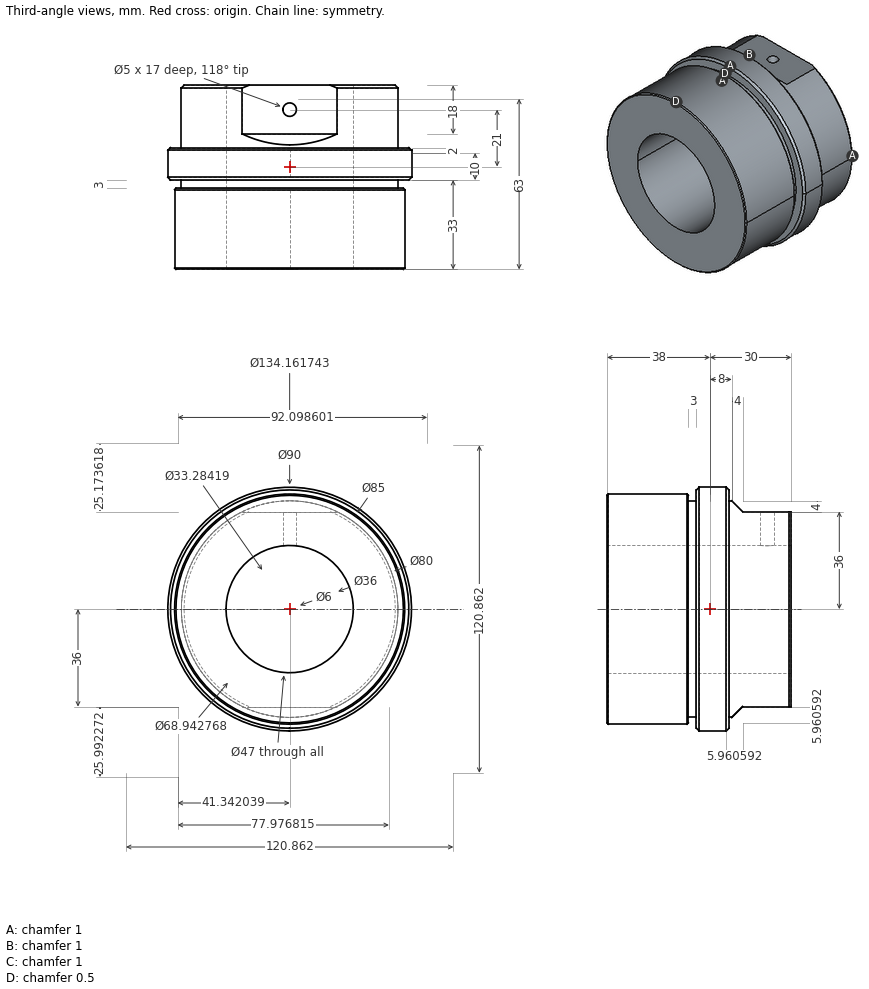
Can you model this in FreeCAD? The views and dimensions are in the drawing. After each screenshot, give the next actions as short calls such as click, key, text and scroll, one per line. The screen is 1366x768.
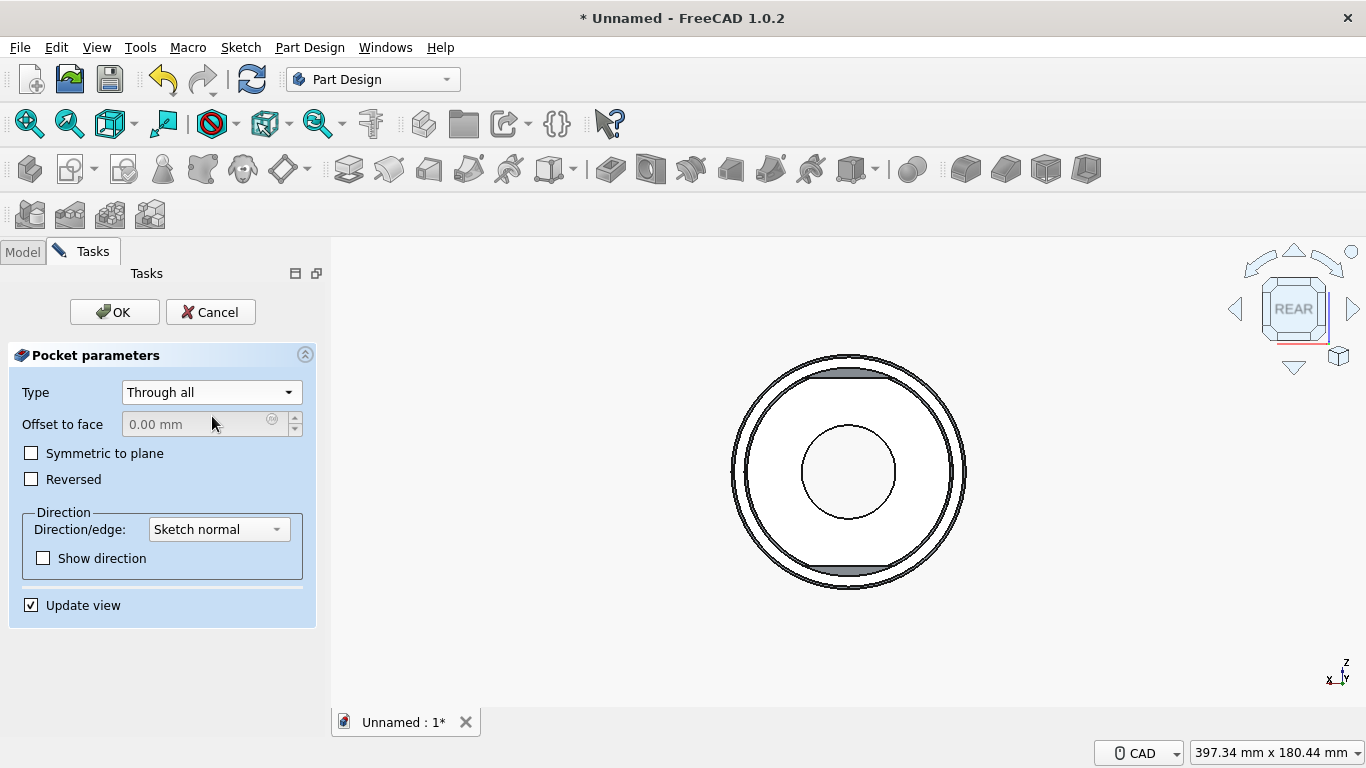
click(30, 479)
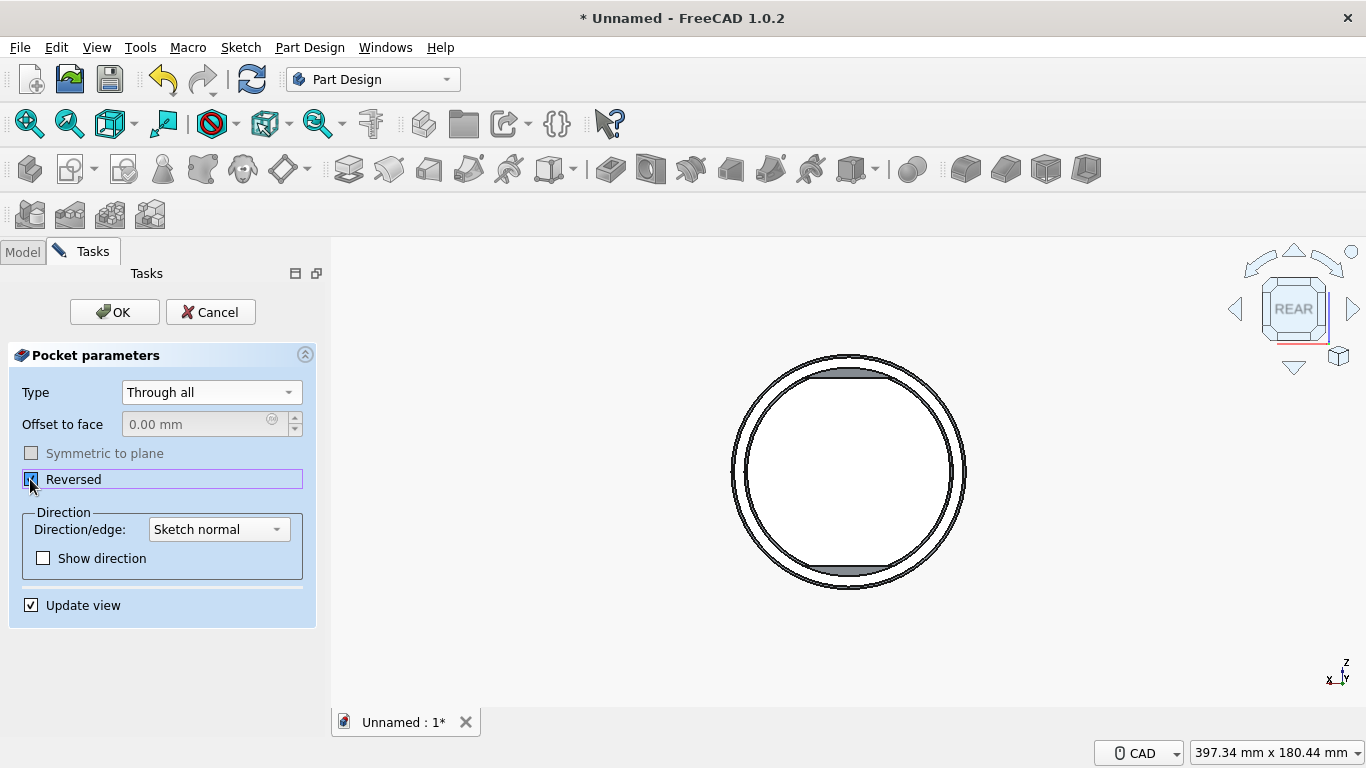
click(115, 312)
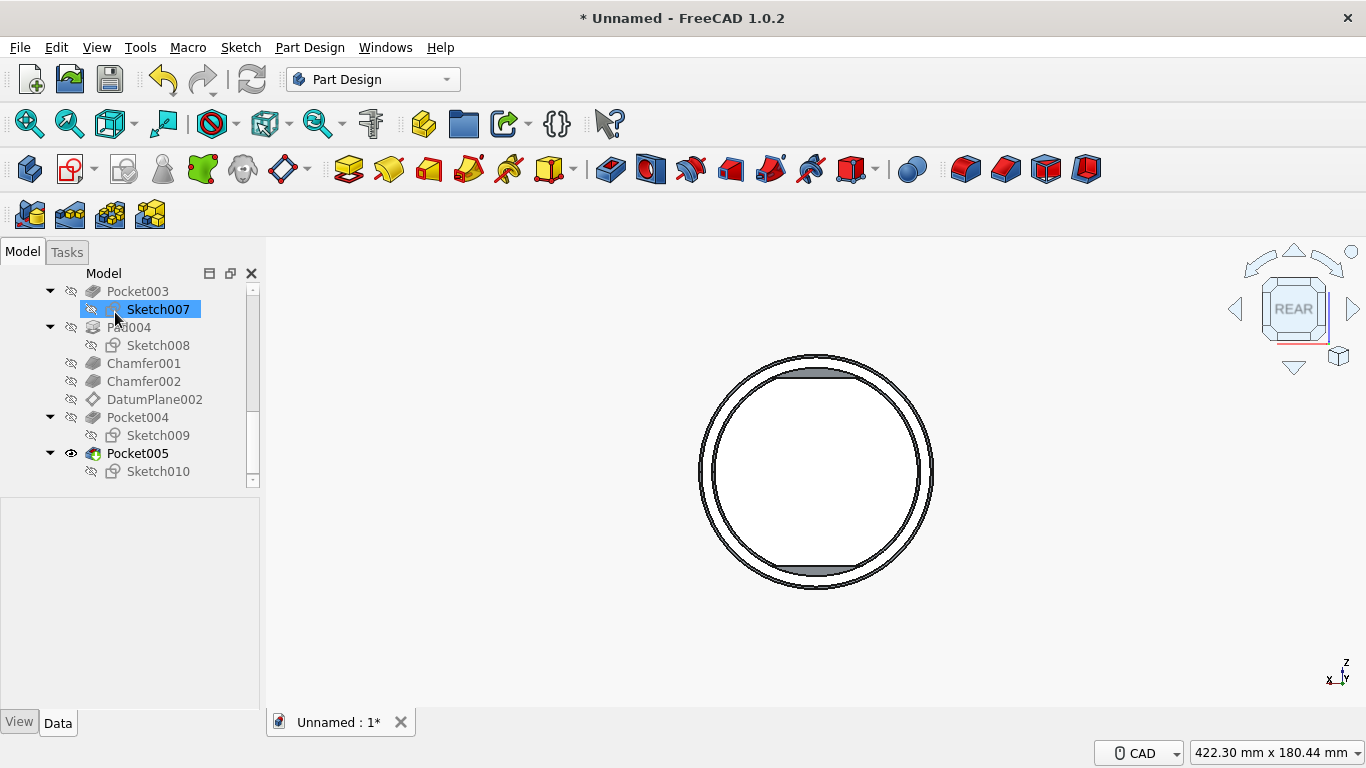
click(816, 471)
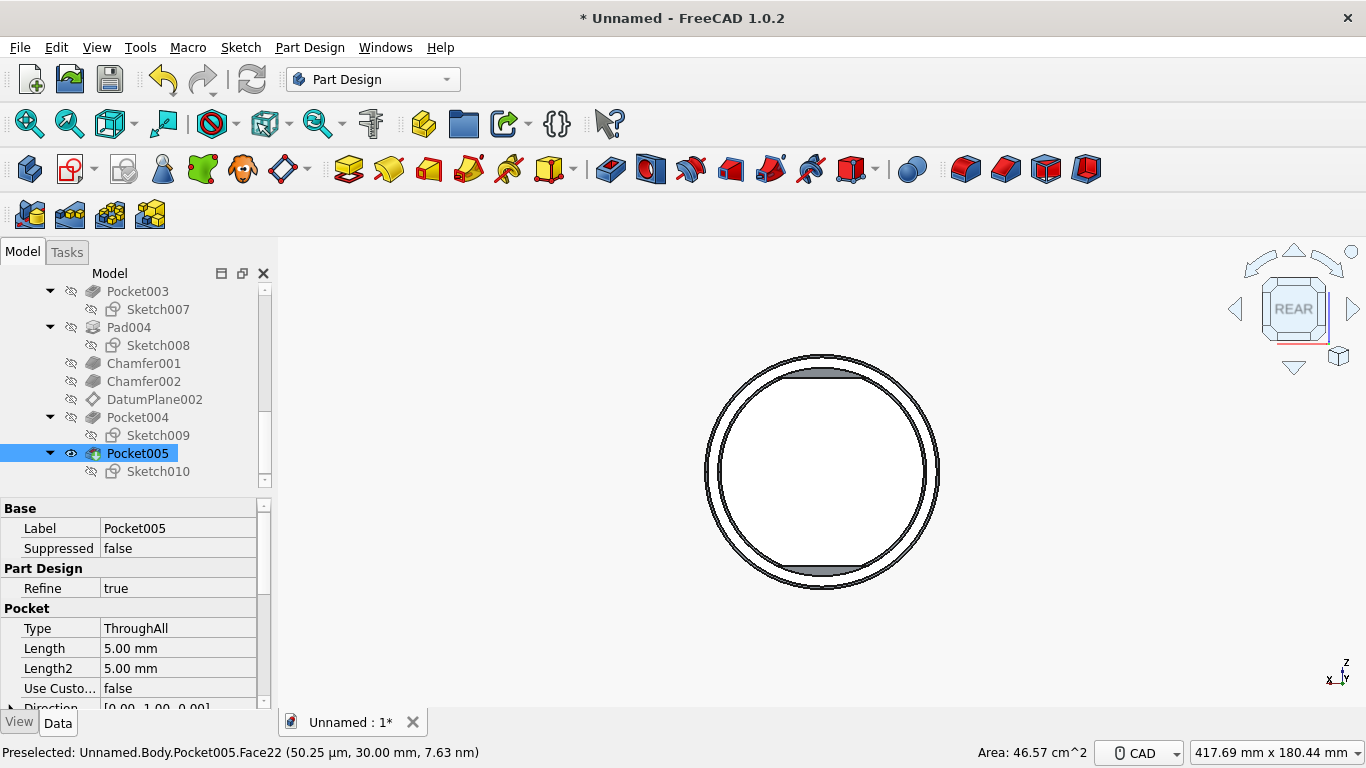
click(70, 170)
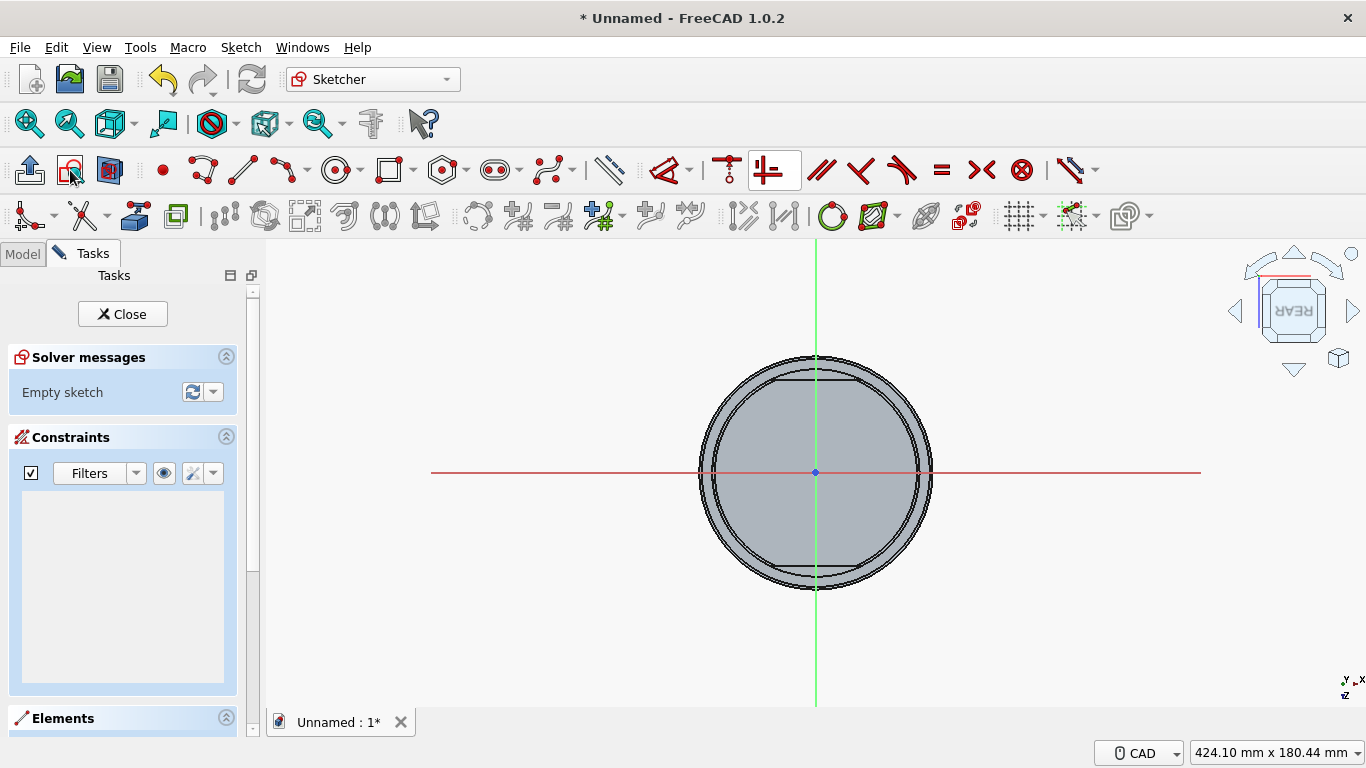
scroll(872, 473, up, 4)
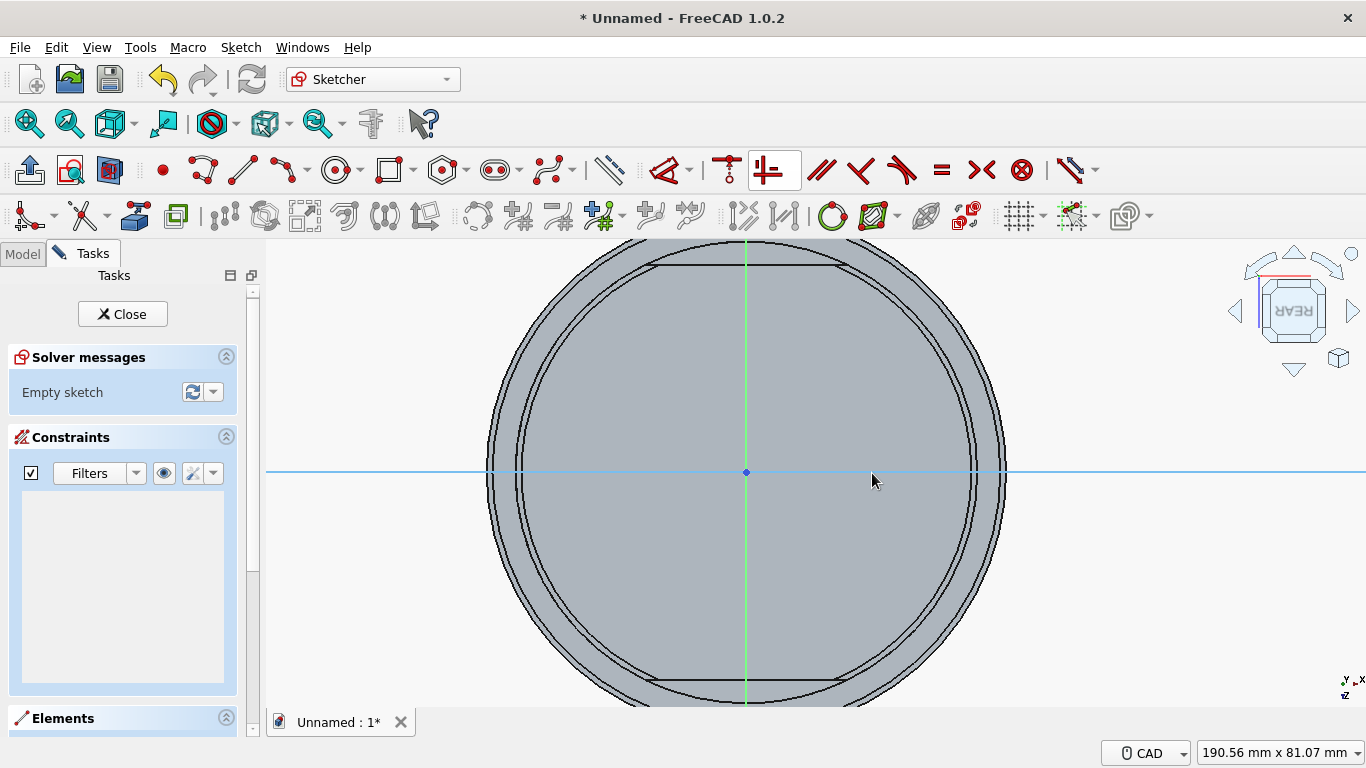
click(336, 170)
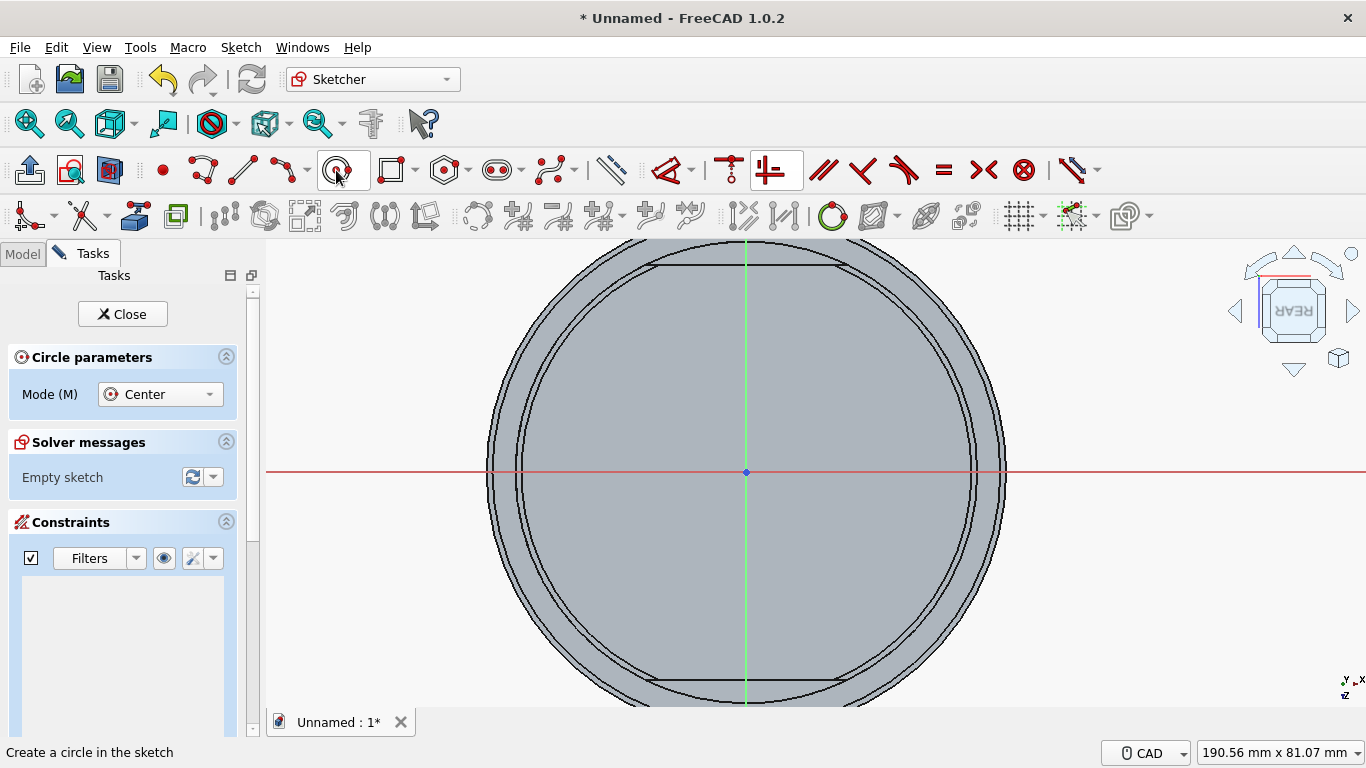
click(746, 472)
click(842, 376)
key(Escape)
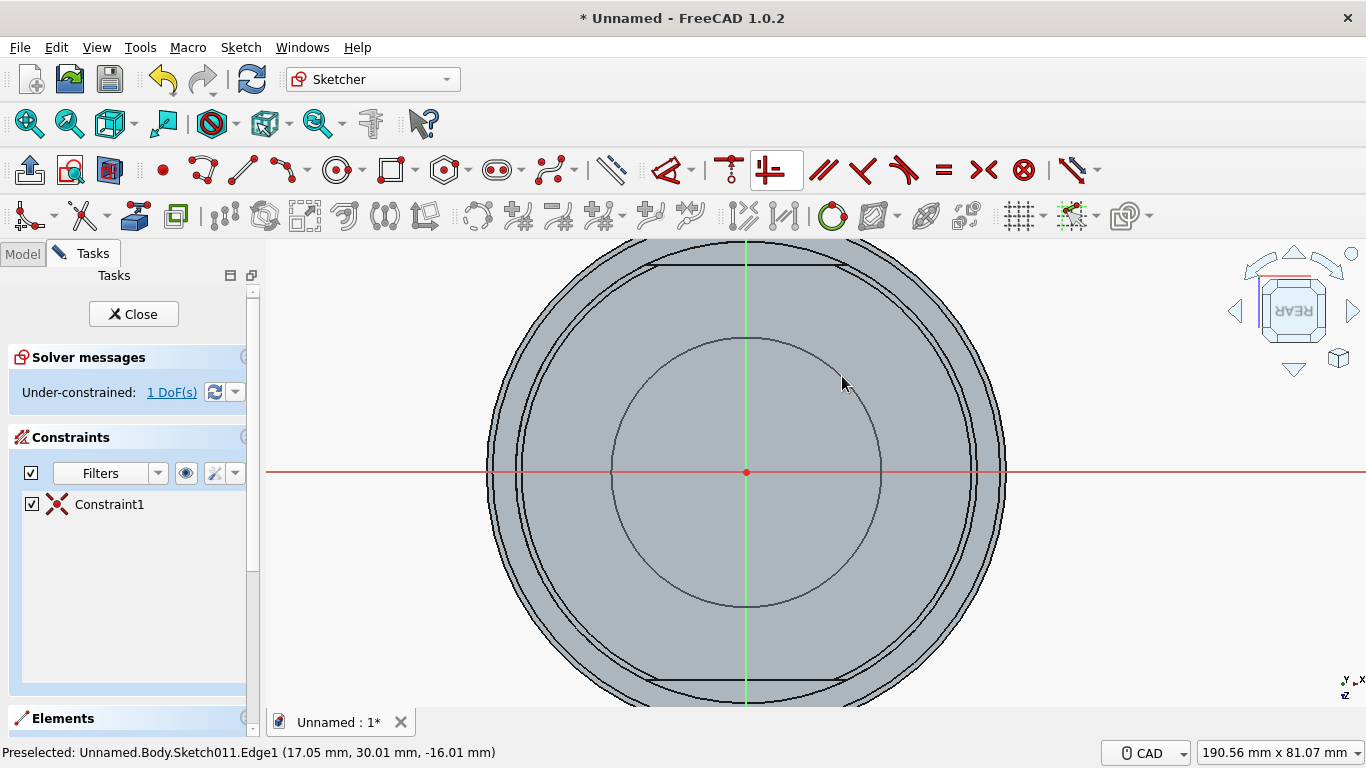
click(666, 170)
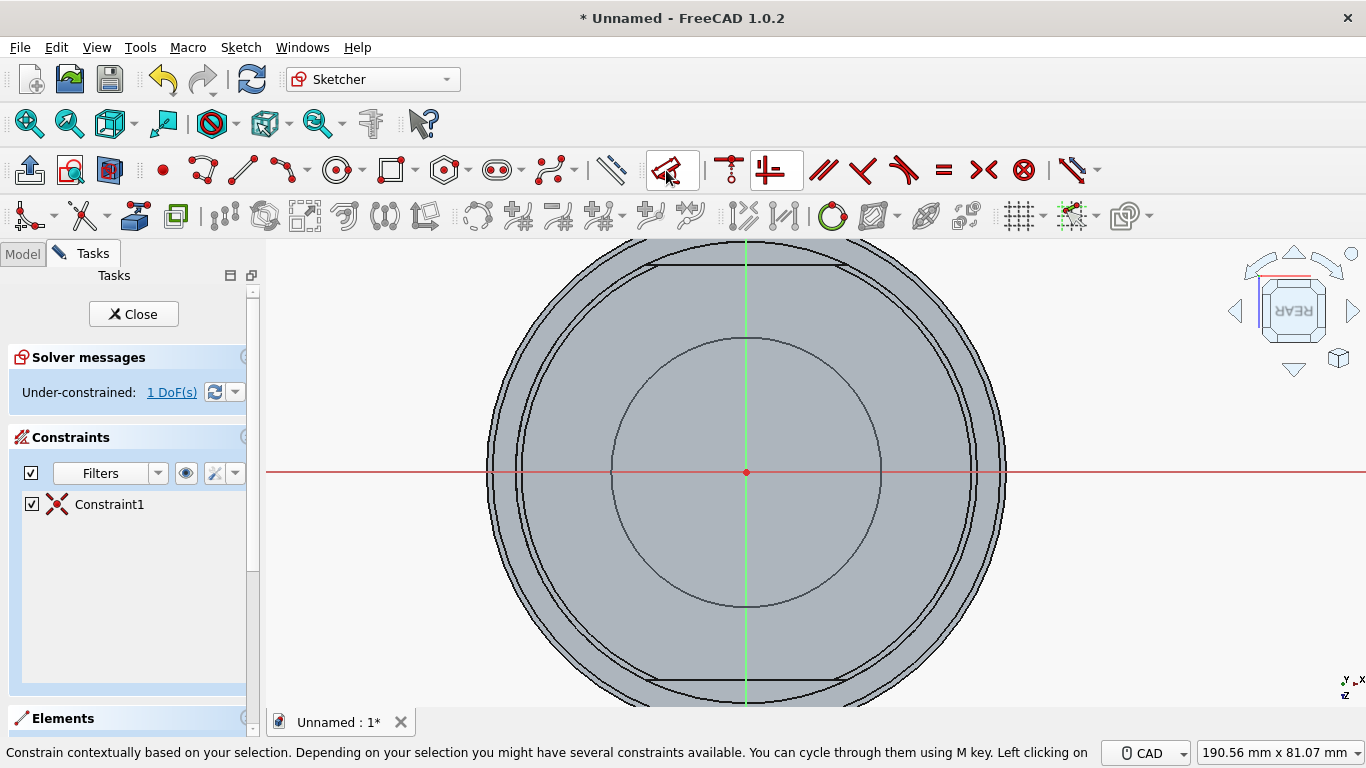
click(842, 377)
click(865, 354)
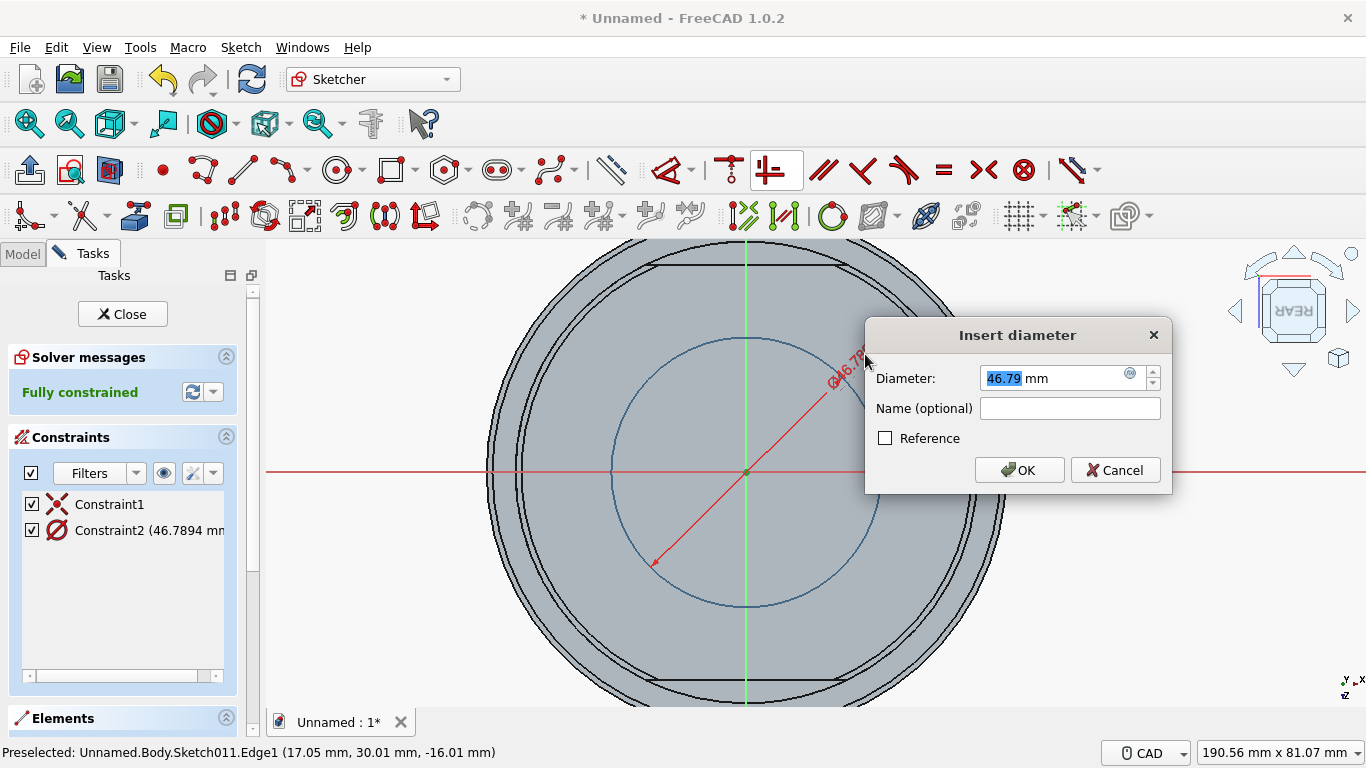
text(47)
key(Return)
key(Escape)